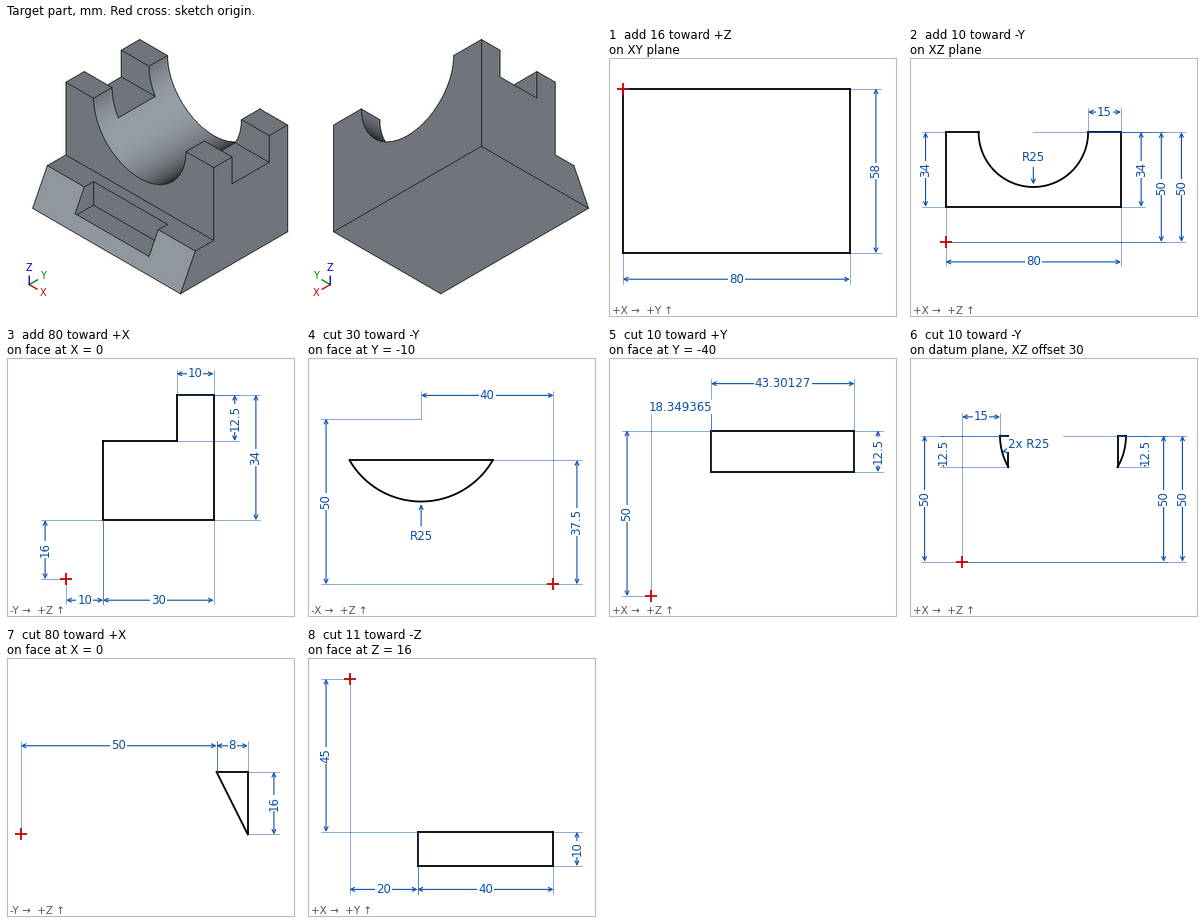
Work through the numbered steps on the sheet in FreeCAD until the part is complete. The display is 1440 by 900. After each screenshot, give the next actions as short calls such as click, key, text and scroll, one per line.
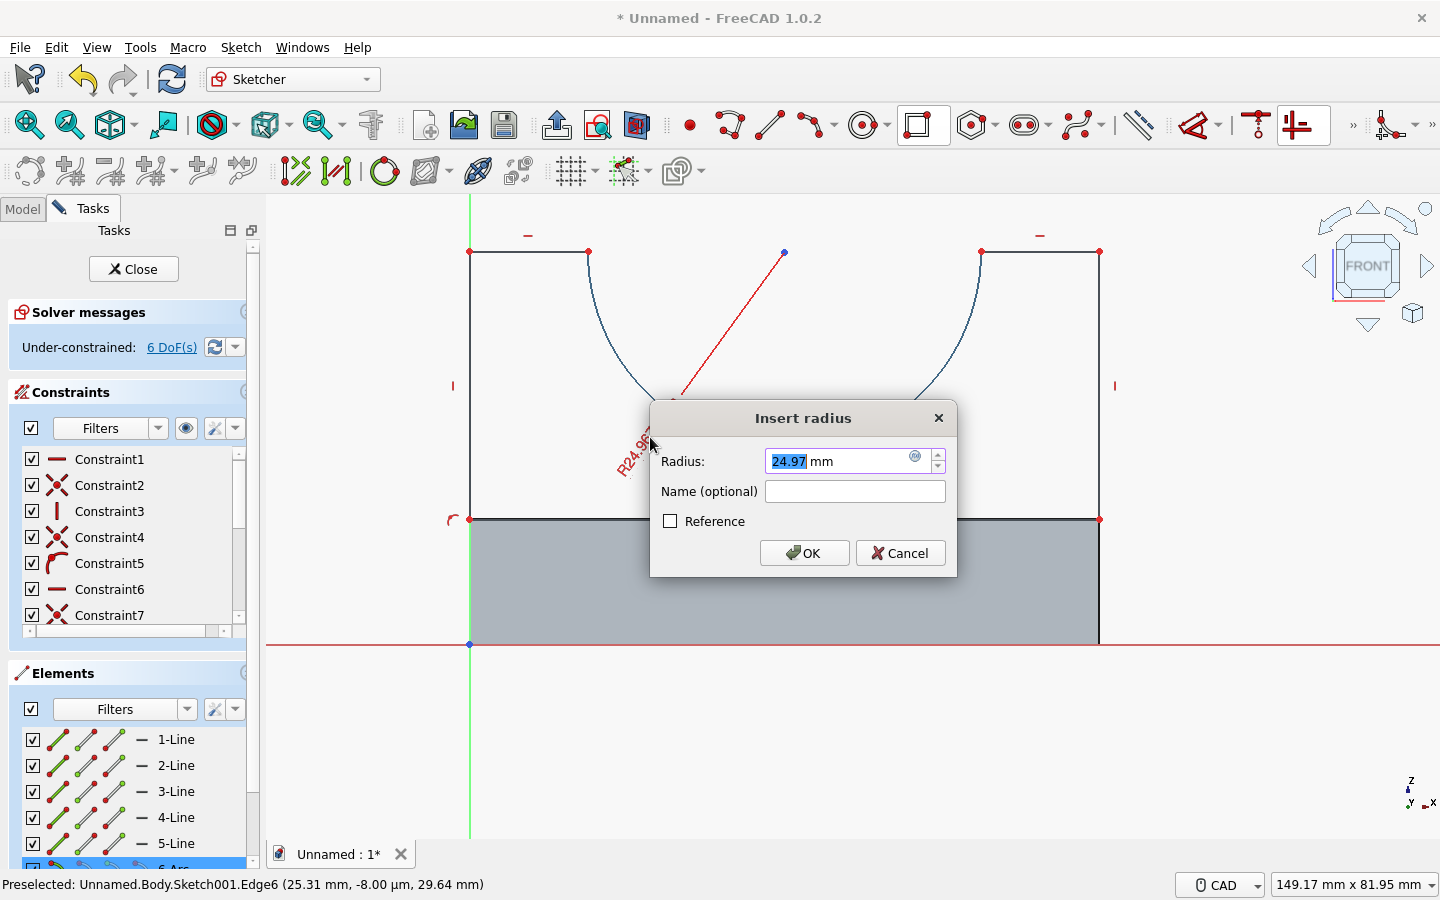
text(25)
key(Return)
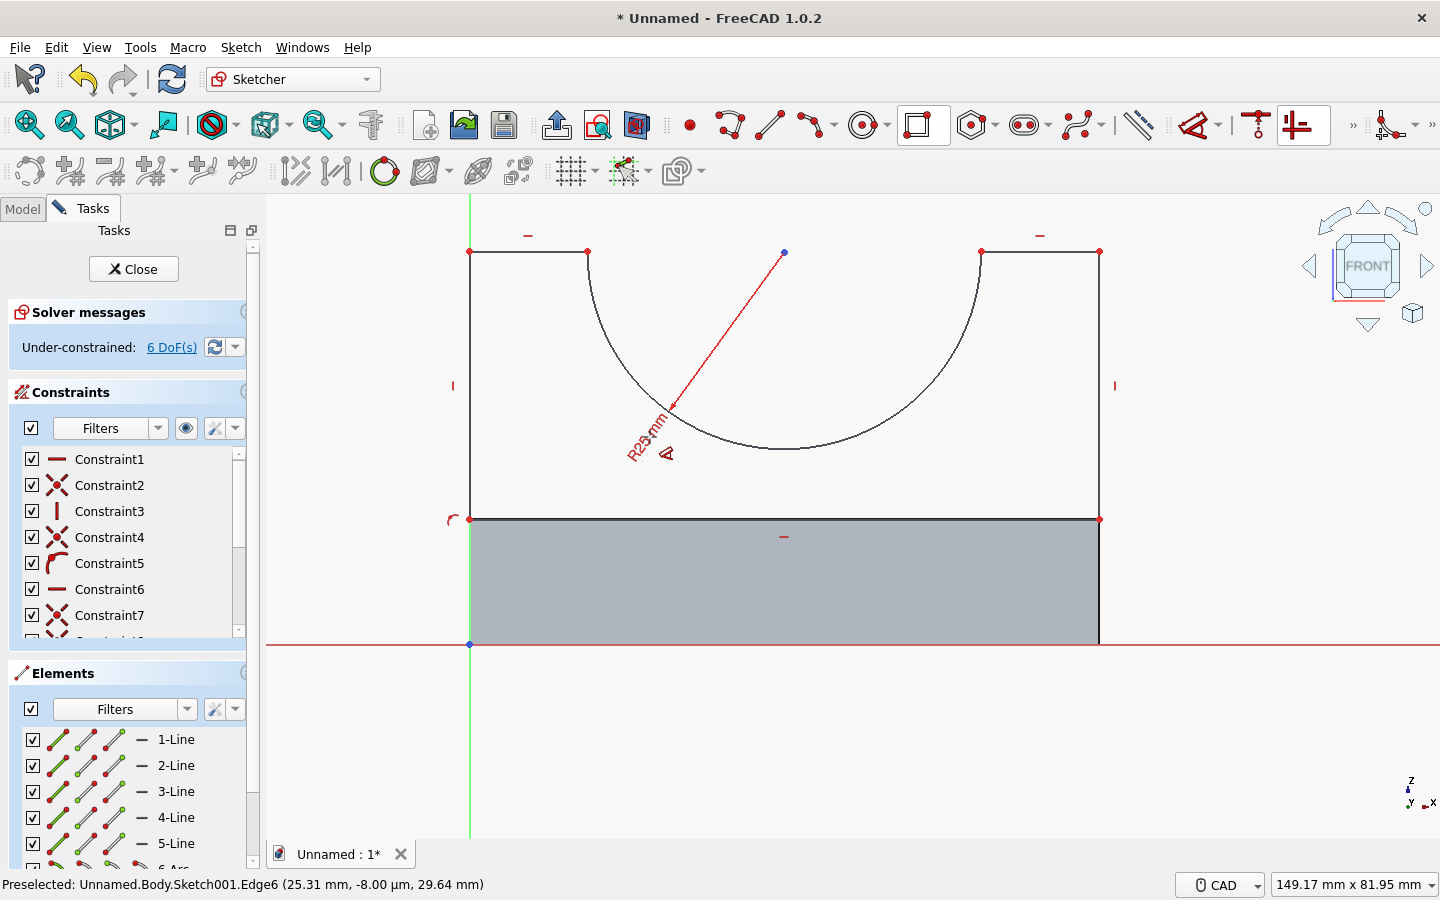
click(1016, 252)
click(1040, 286)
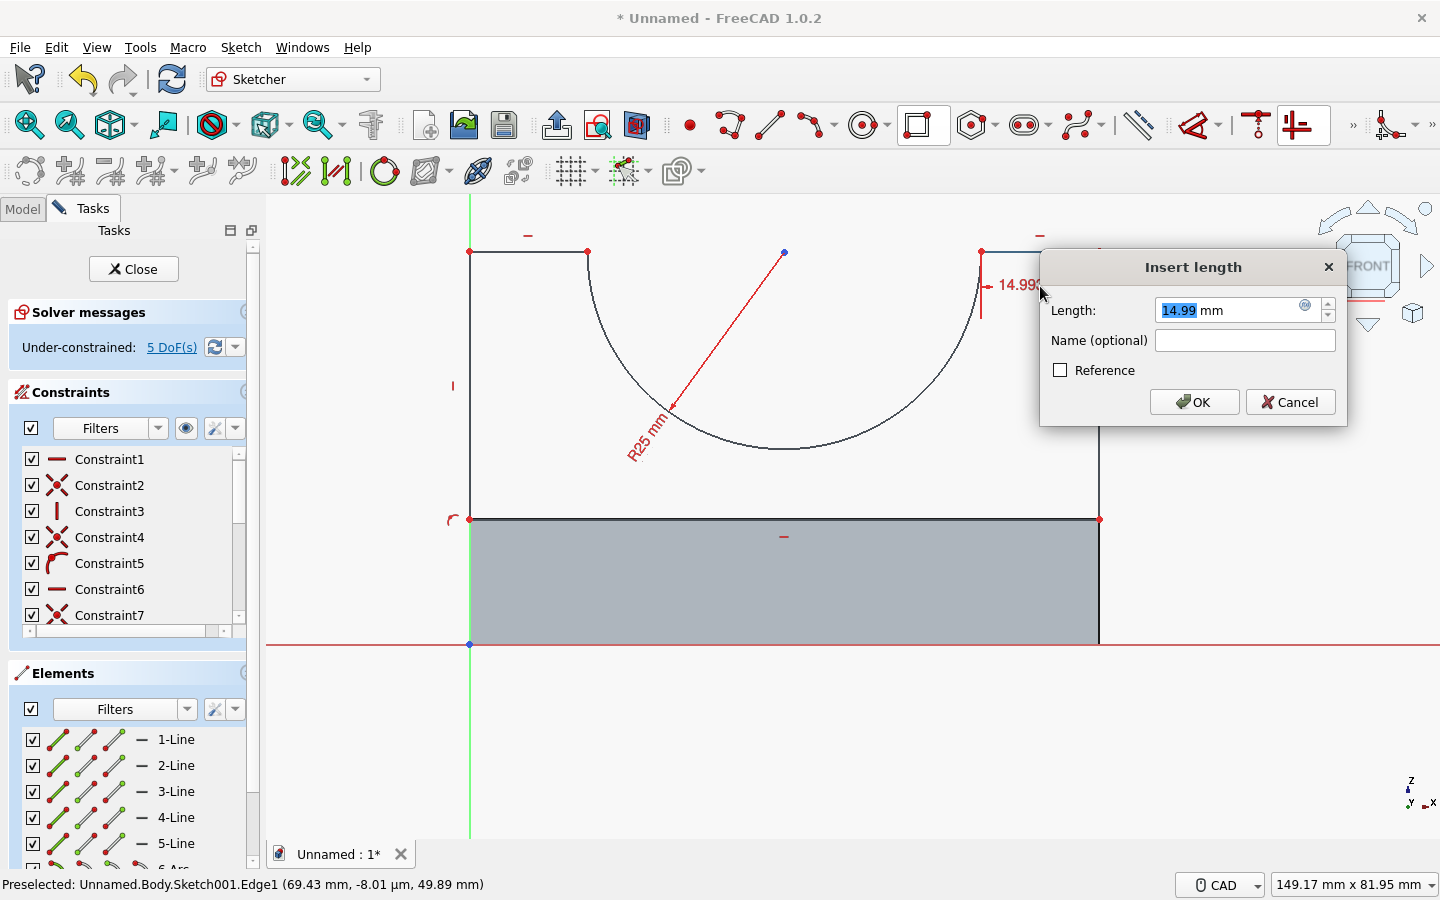
text(15)
key(Return)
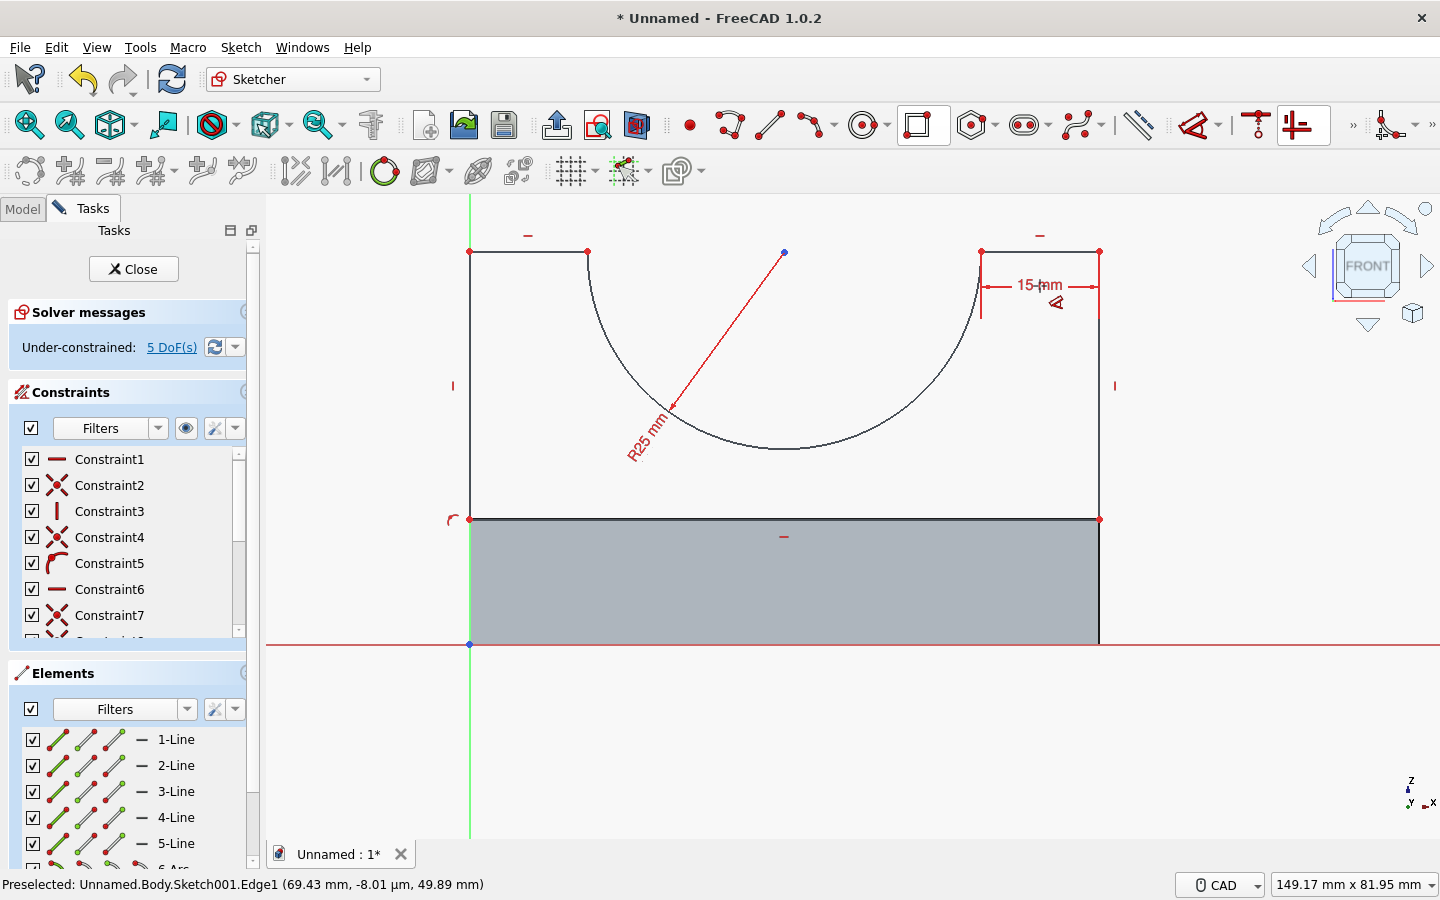
click(1099, 332)
click(1133, 386)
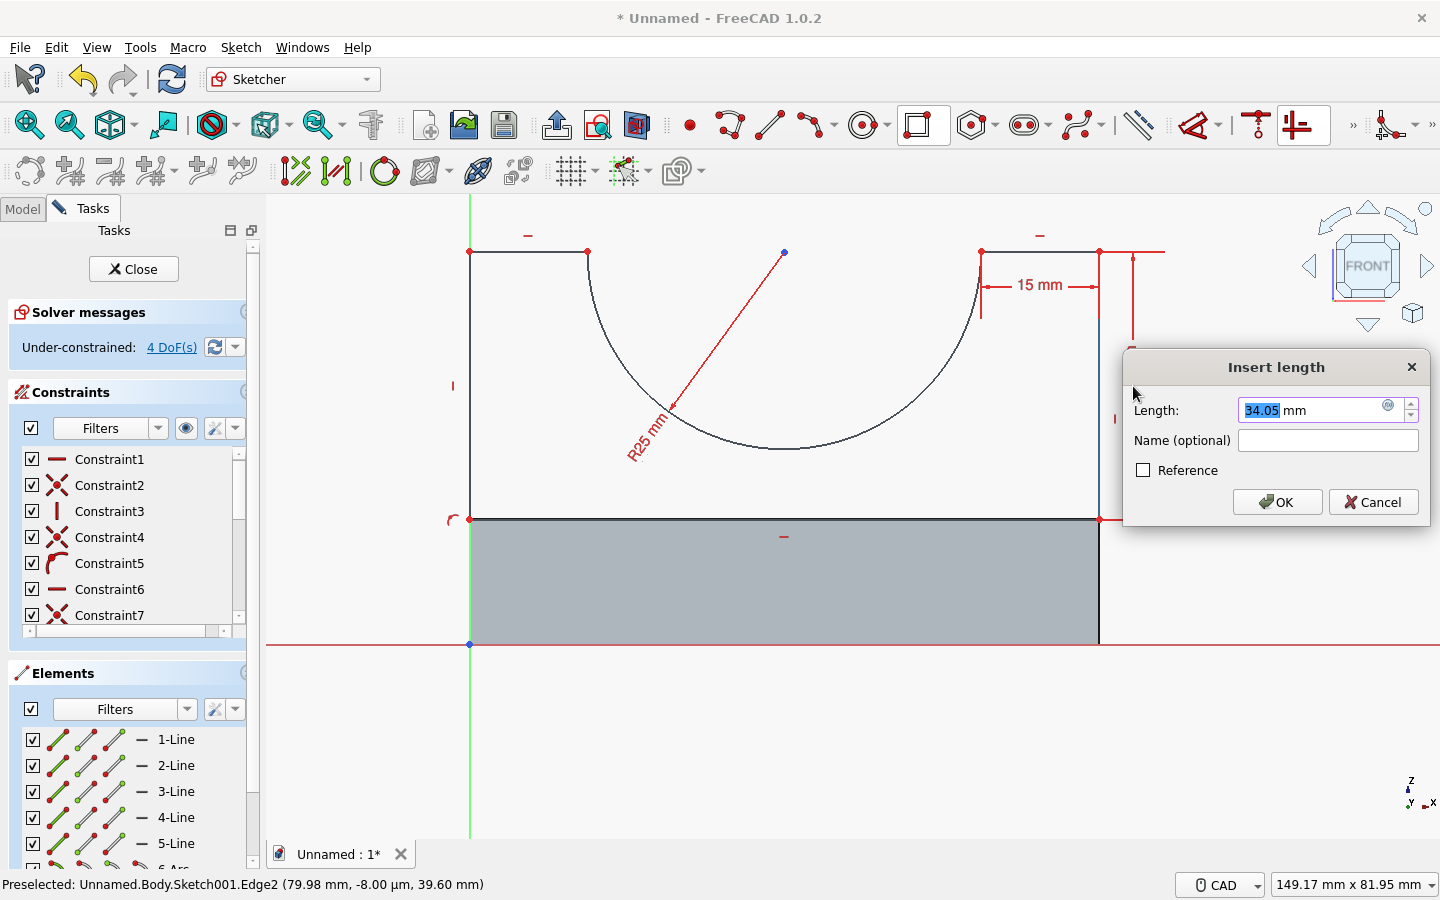
text(34)
key(Return)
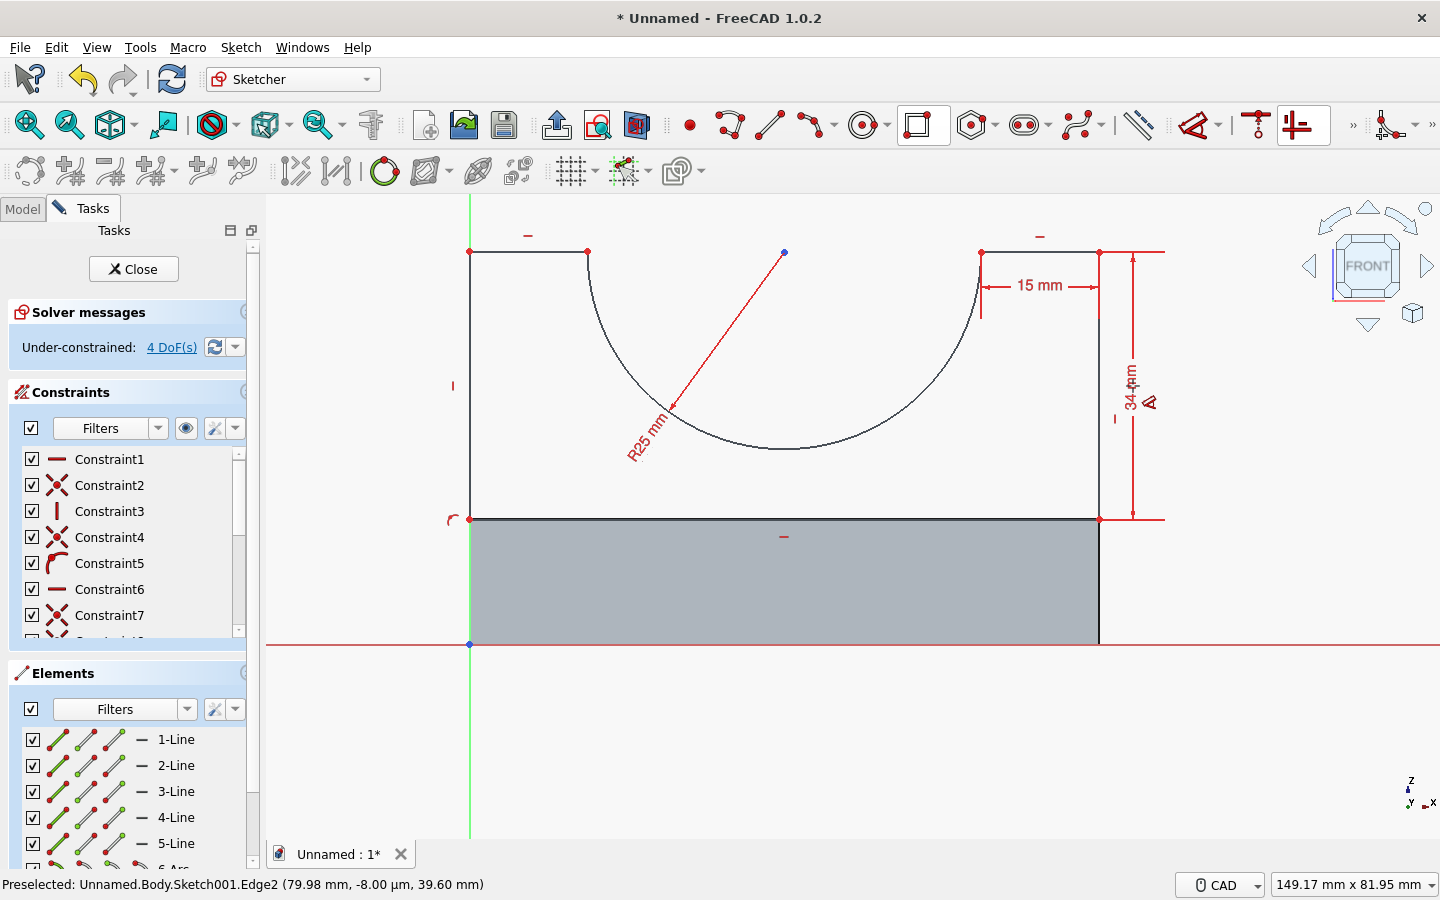
click(910, 520)
click(784, 554)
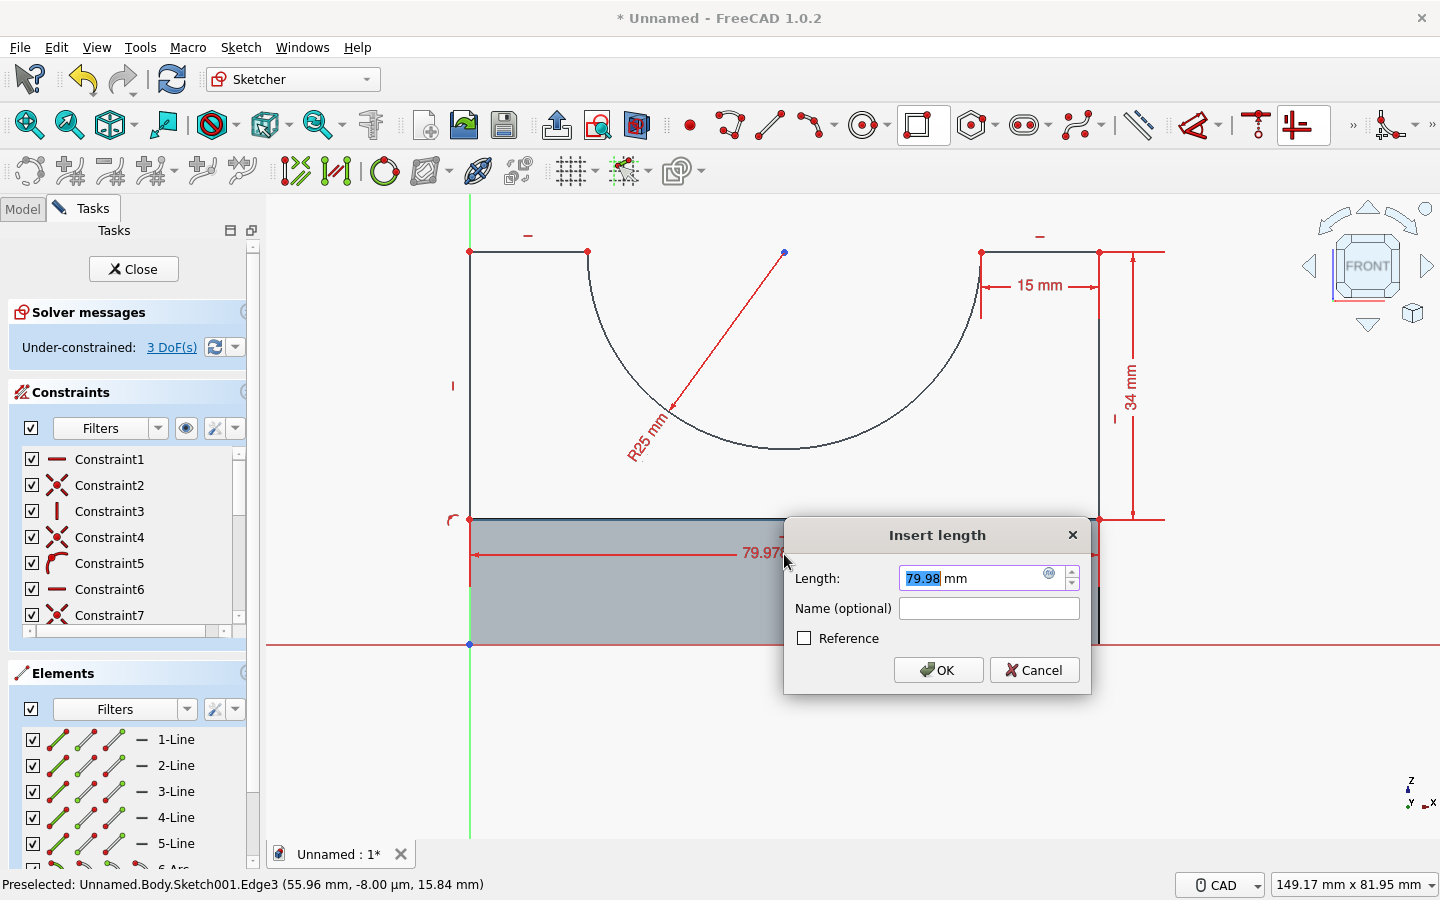
text(80)
key(Return)